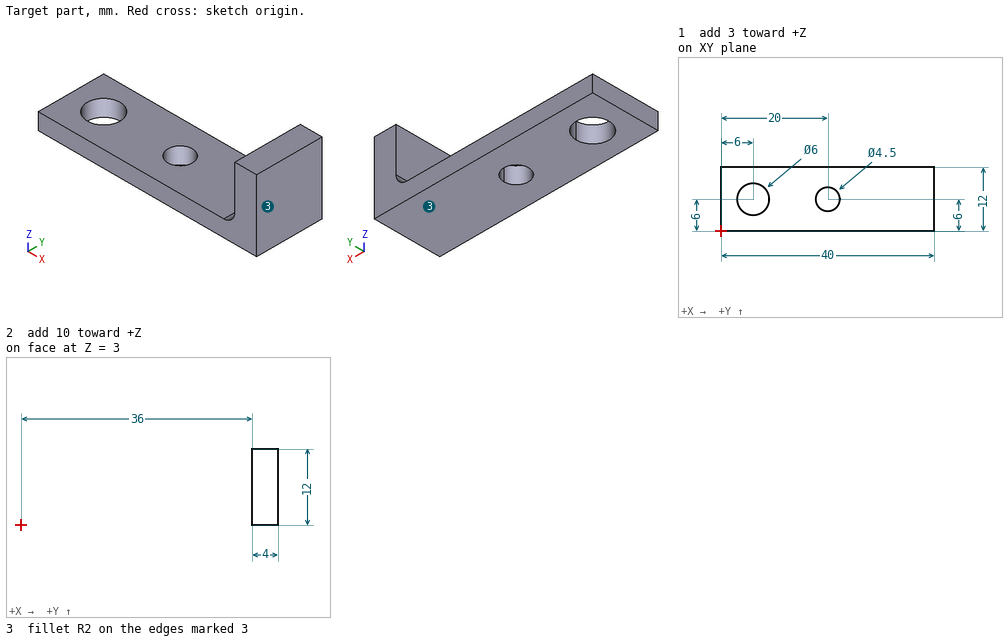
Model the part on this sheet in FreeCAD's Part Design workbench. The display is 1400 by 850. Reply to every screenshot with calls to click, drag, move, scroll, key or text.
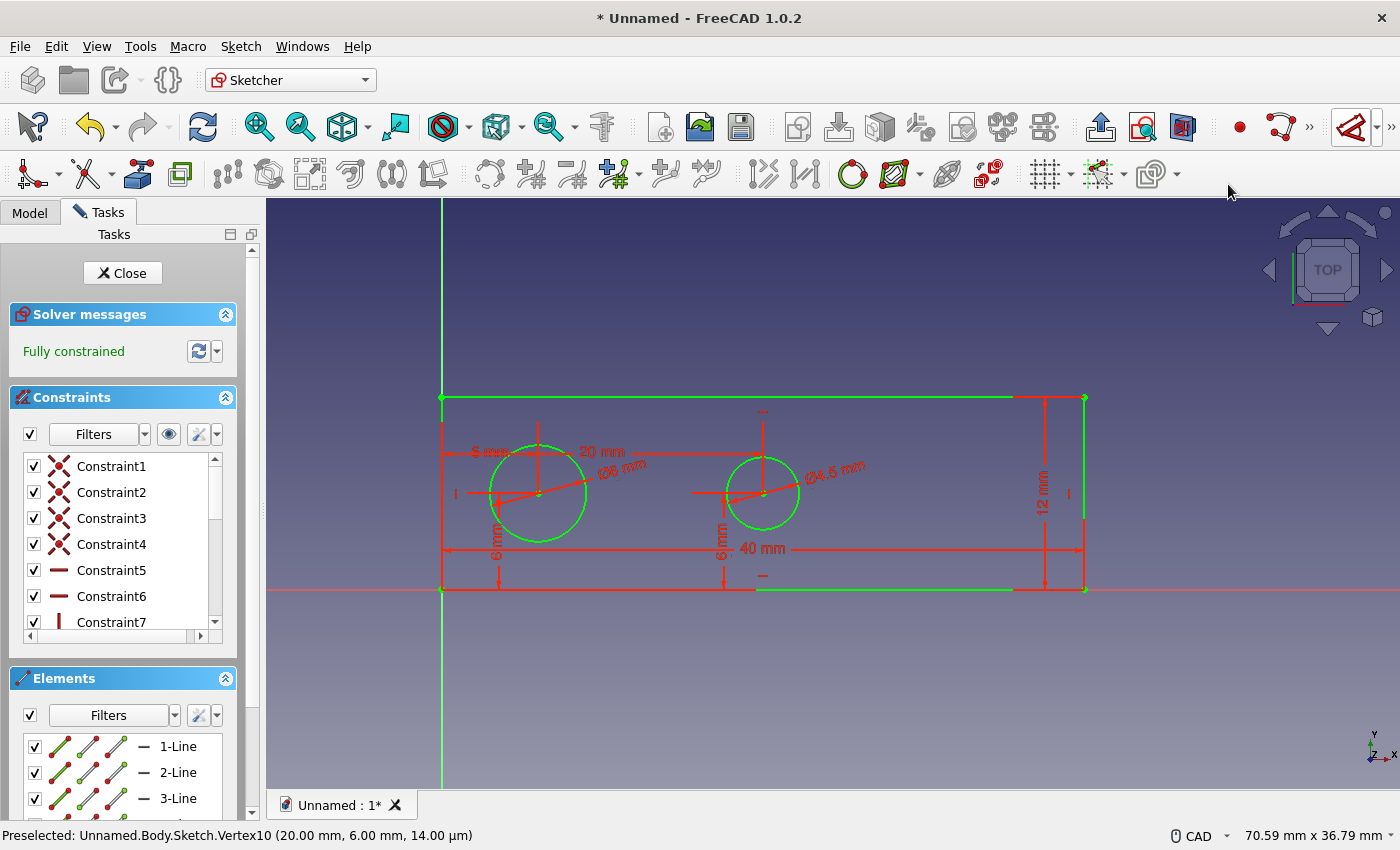
click(123, 273)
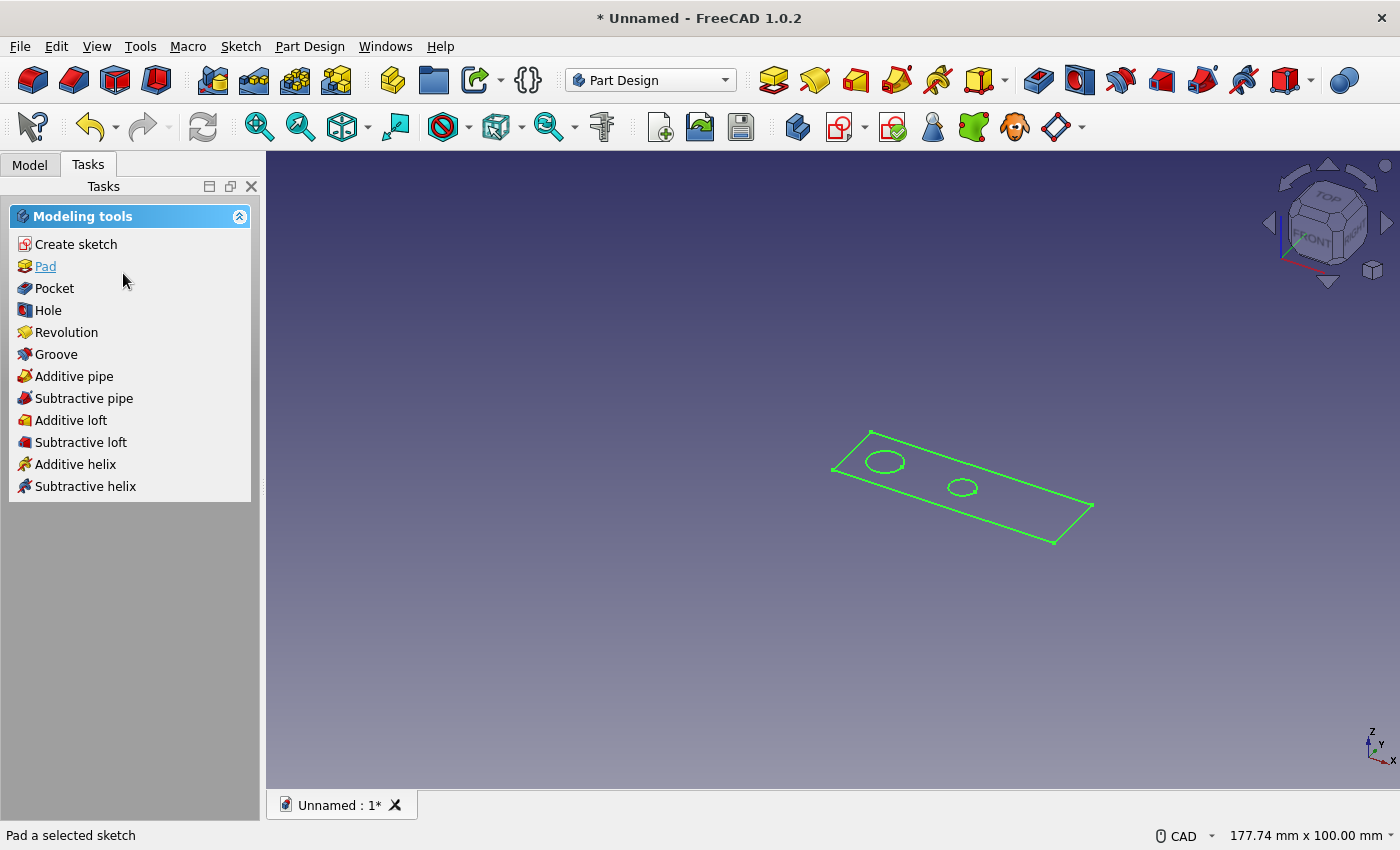
click(774, 80)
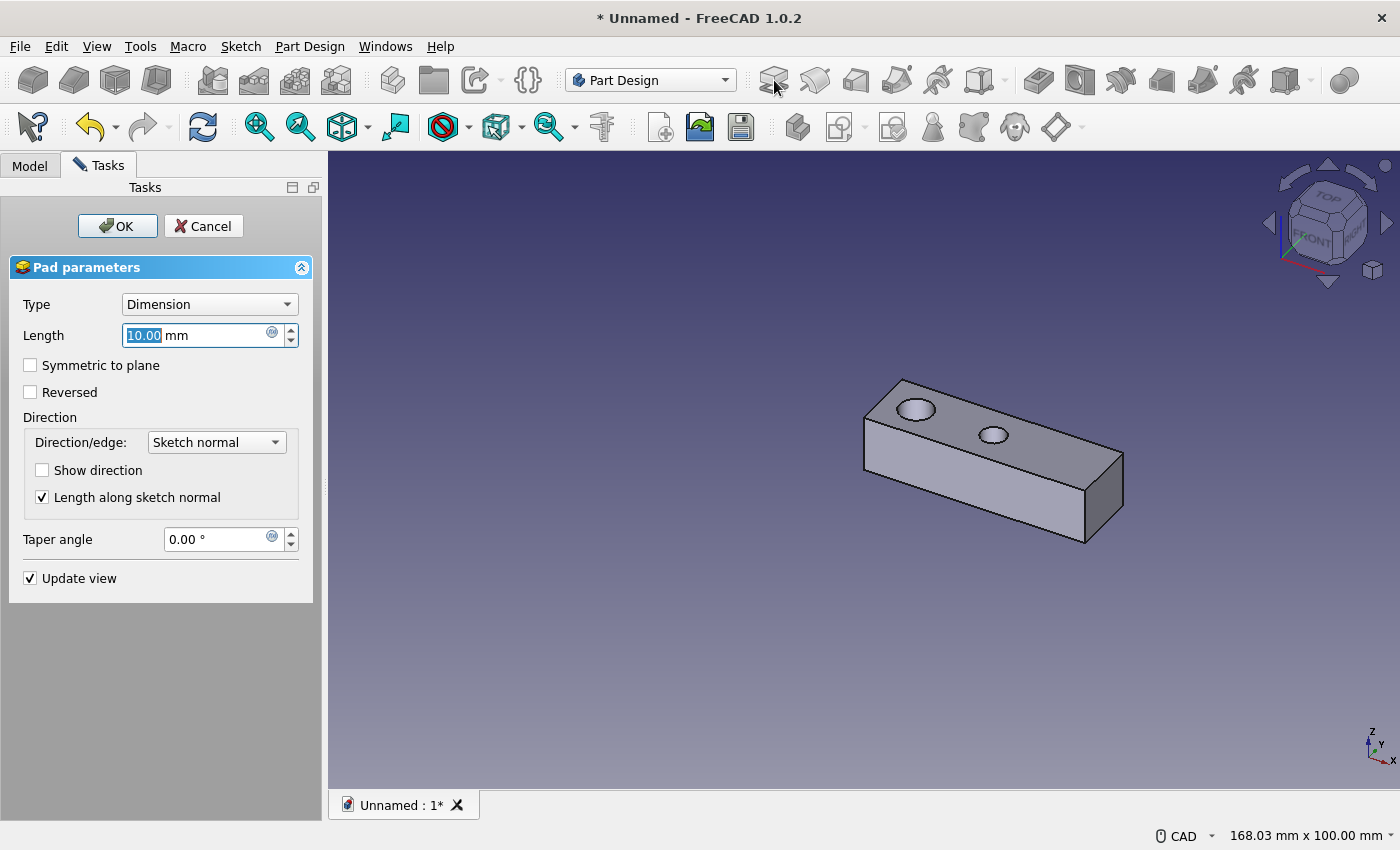
text(3)
key(Tab)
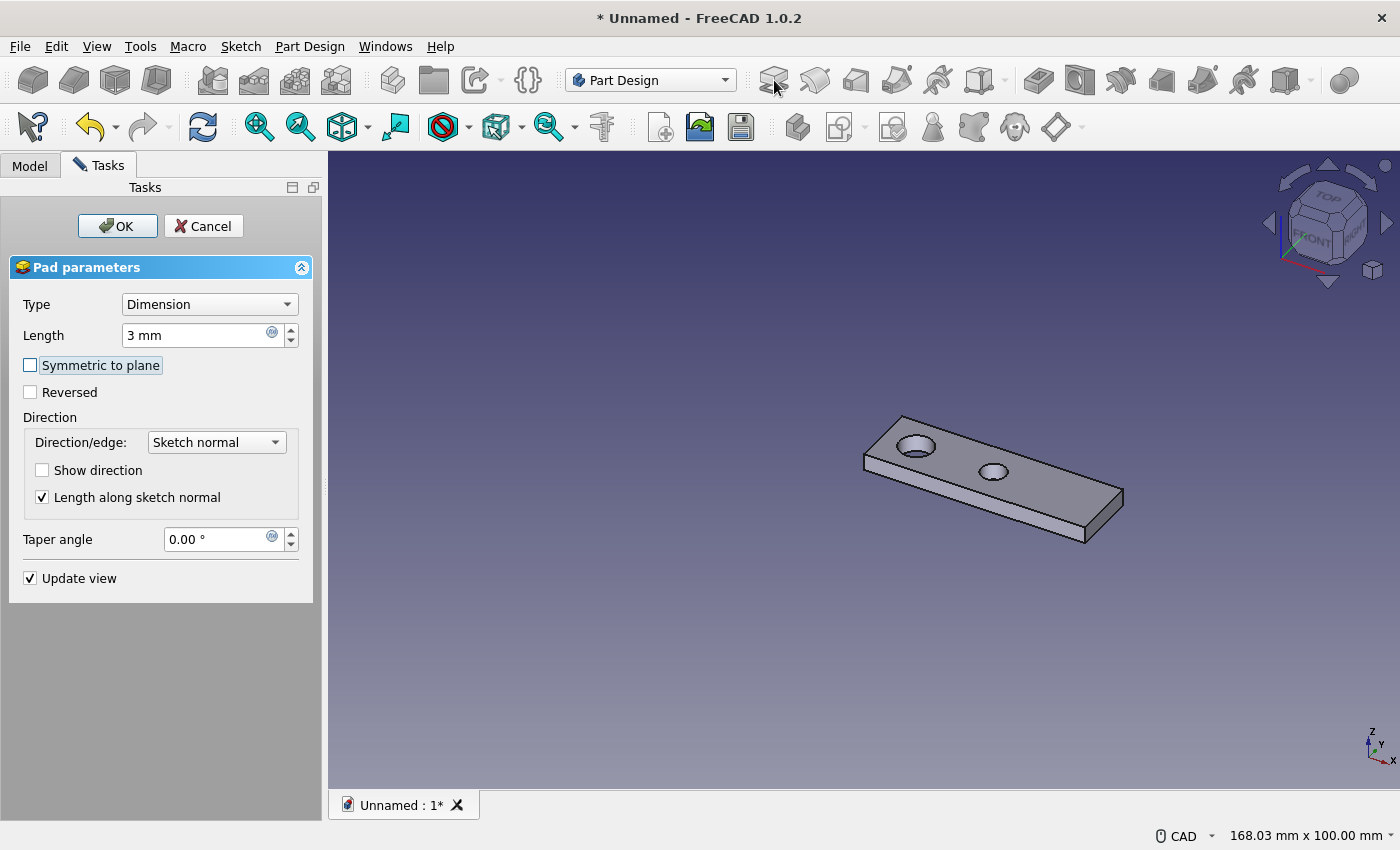
click(118, 226)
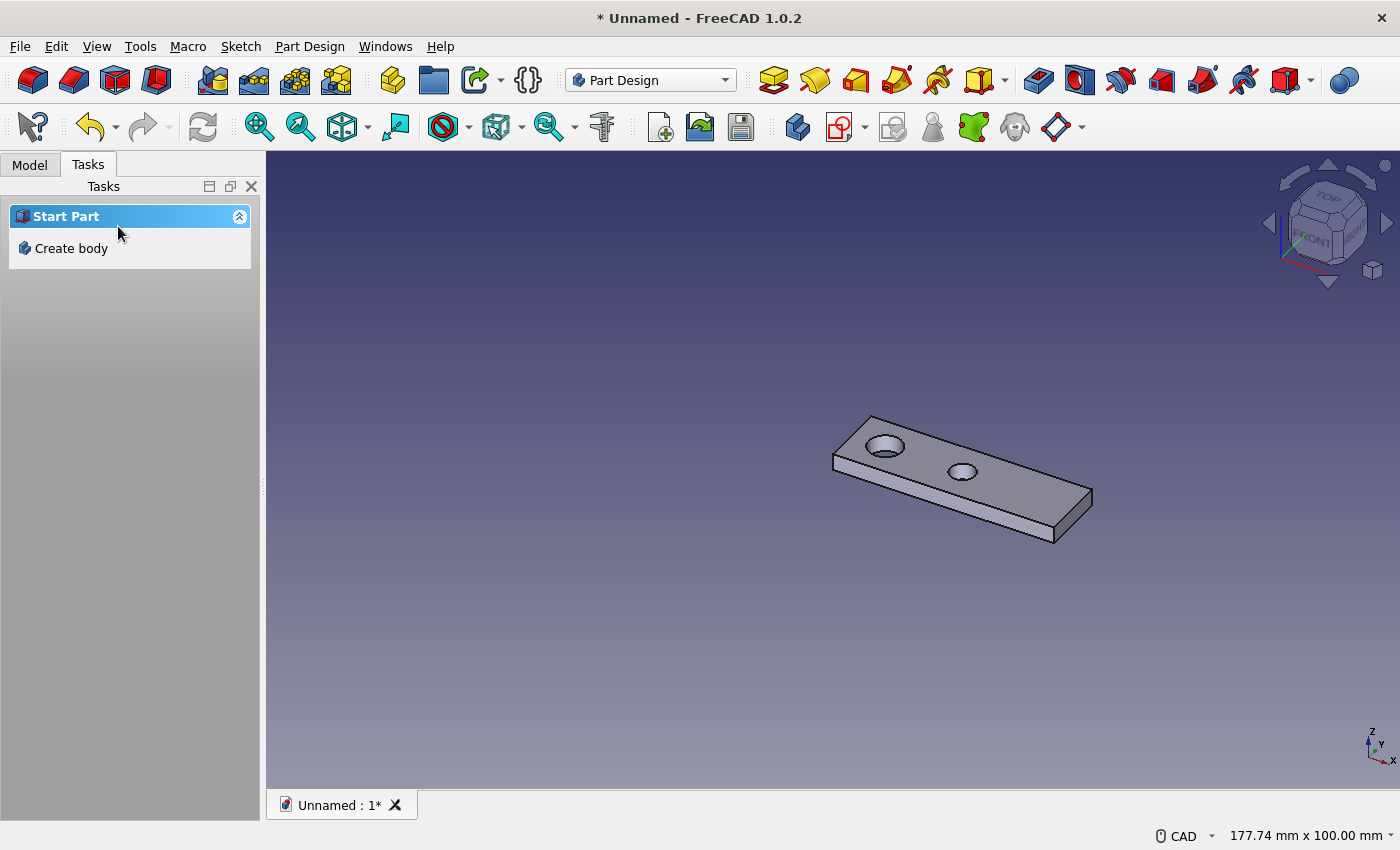
click(260, 128)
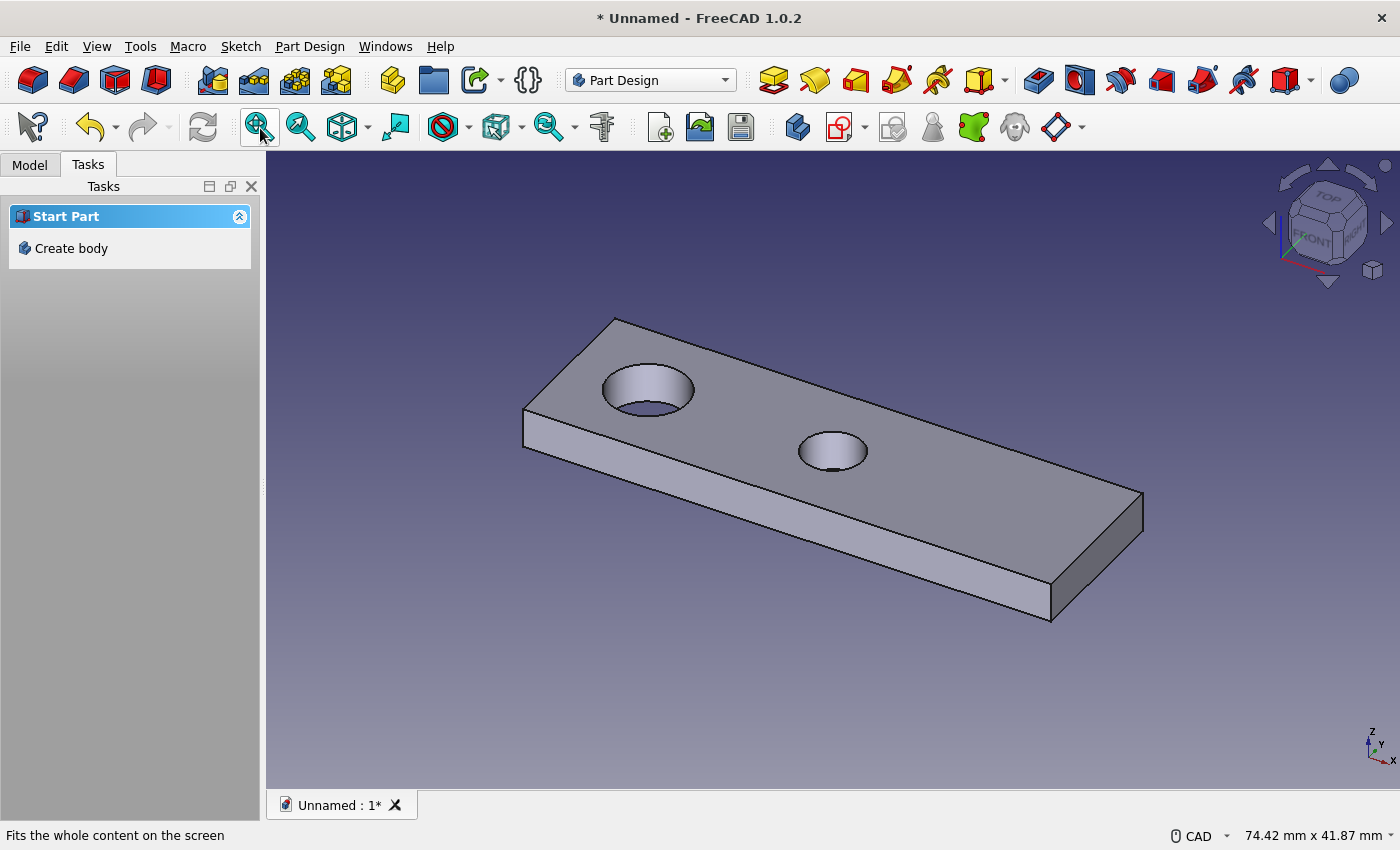
click(984, 500)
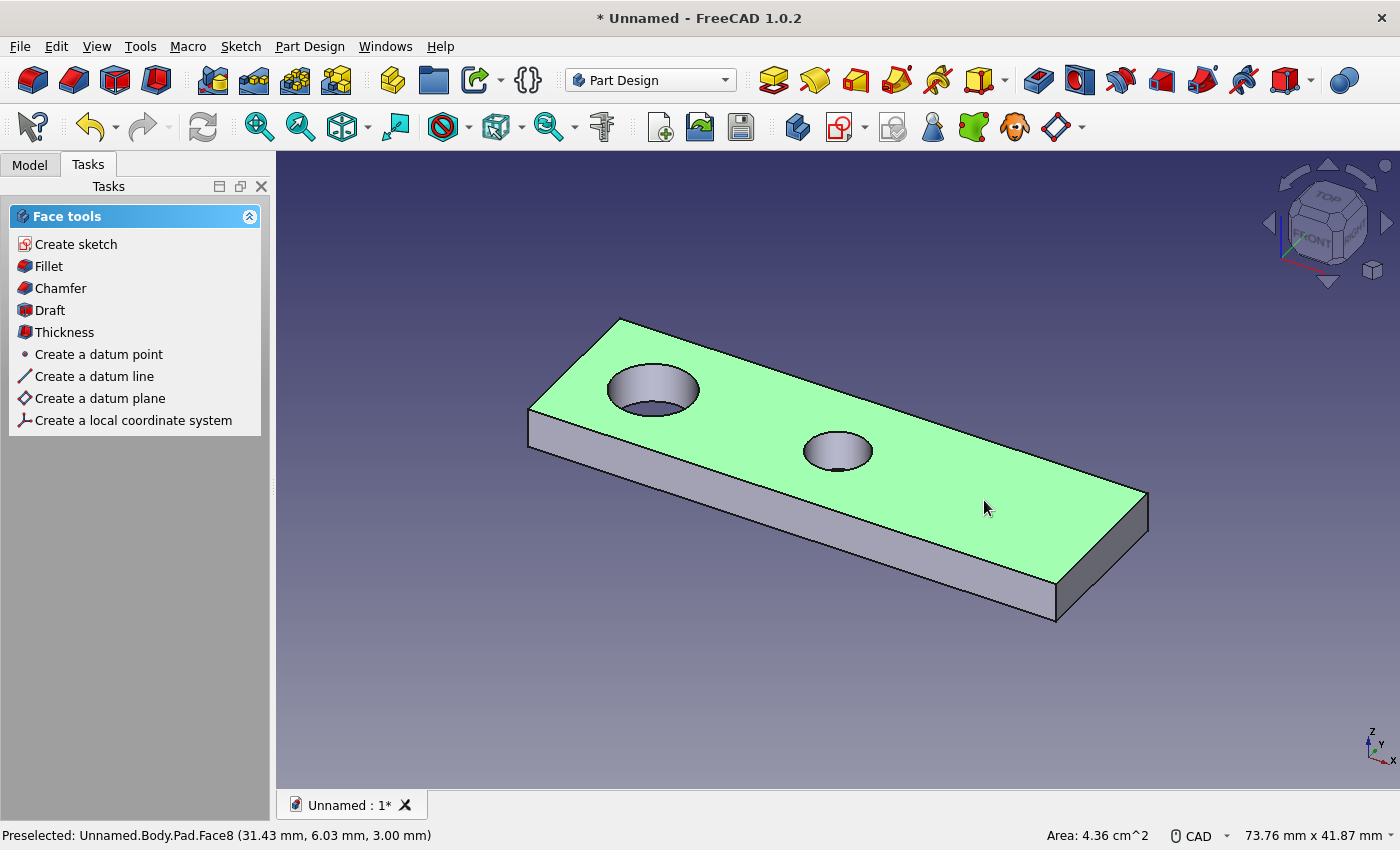
click(838, 128)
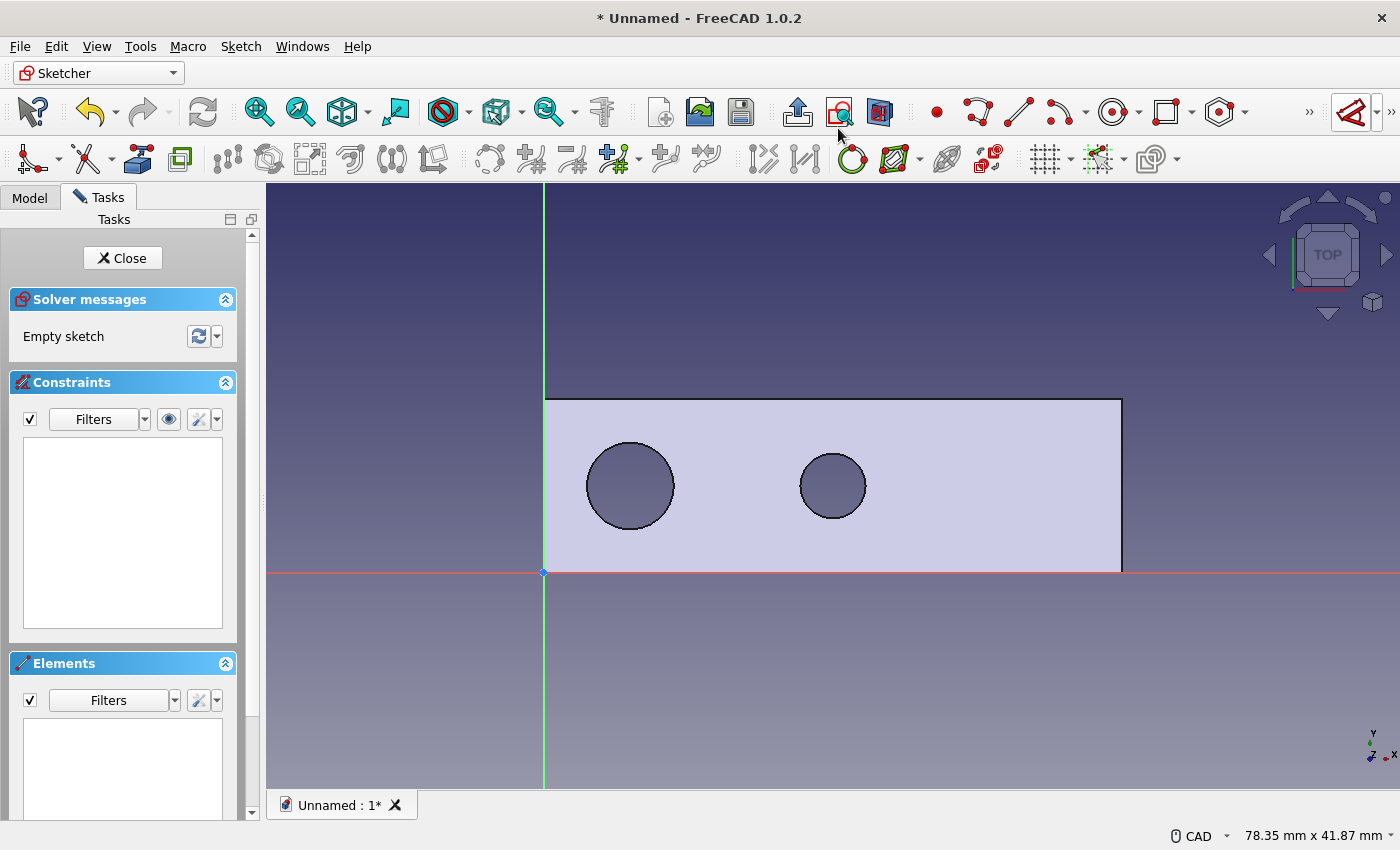
scroll(1235, 486, up, 4)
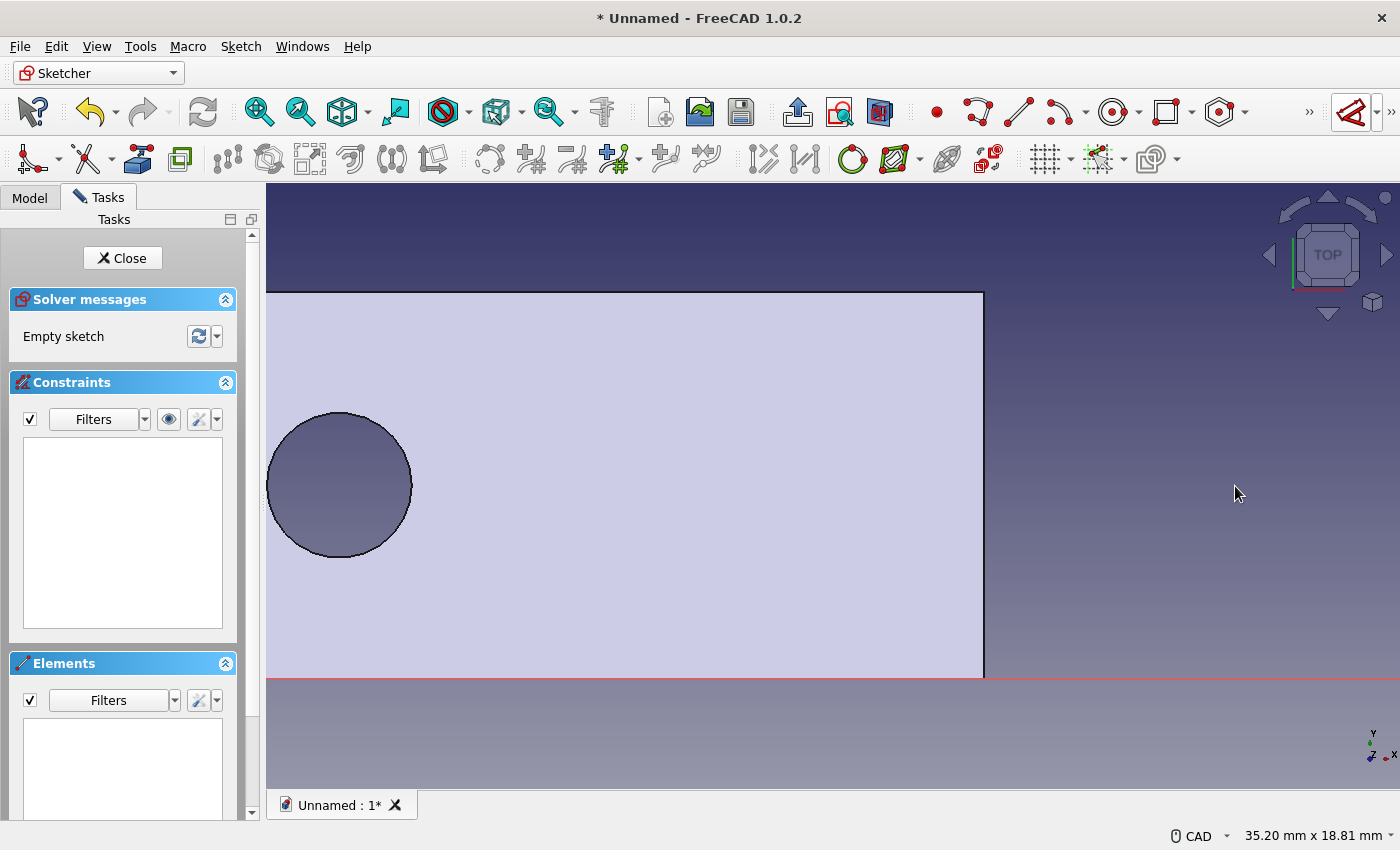
key(g)
key(r)